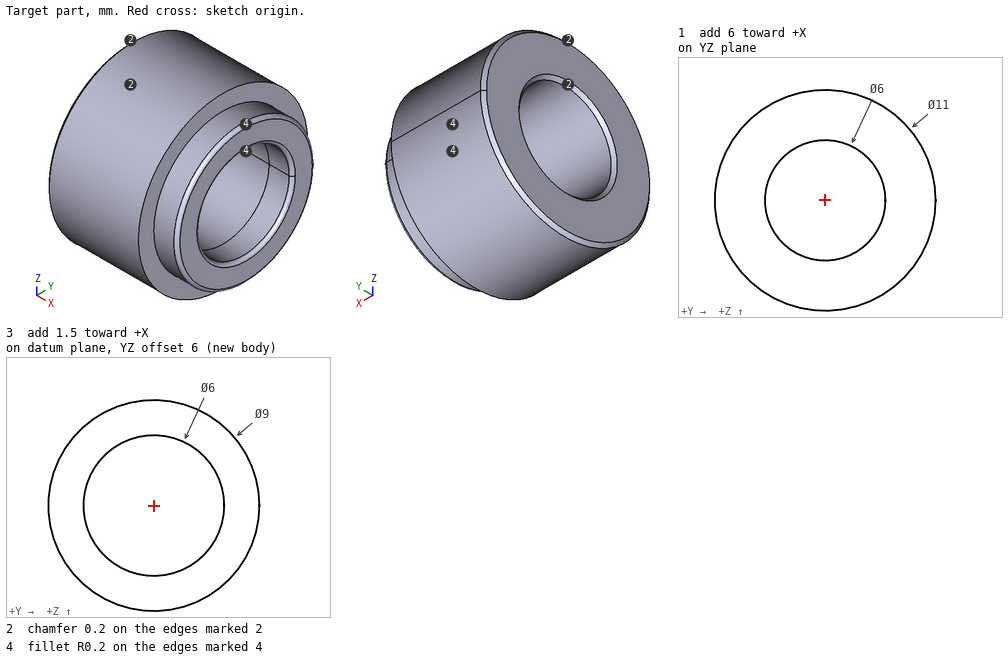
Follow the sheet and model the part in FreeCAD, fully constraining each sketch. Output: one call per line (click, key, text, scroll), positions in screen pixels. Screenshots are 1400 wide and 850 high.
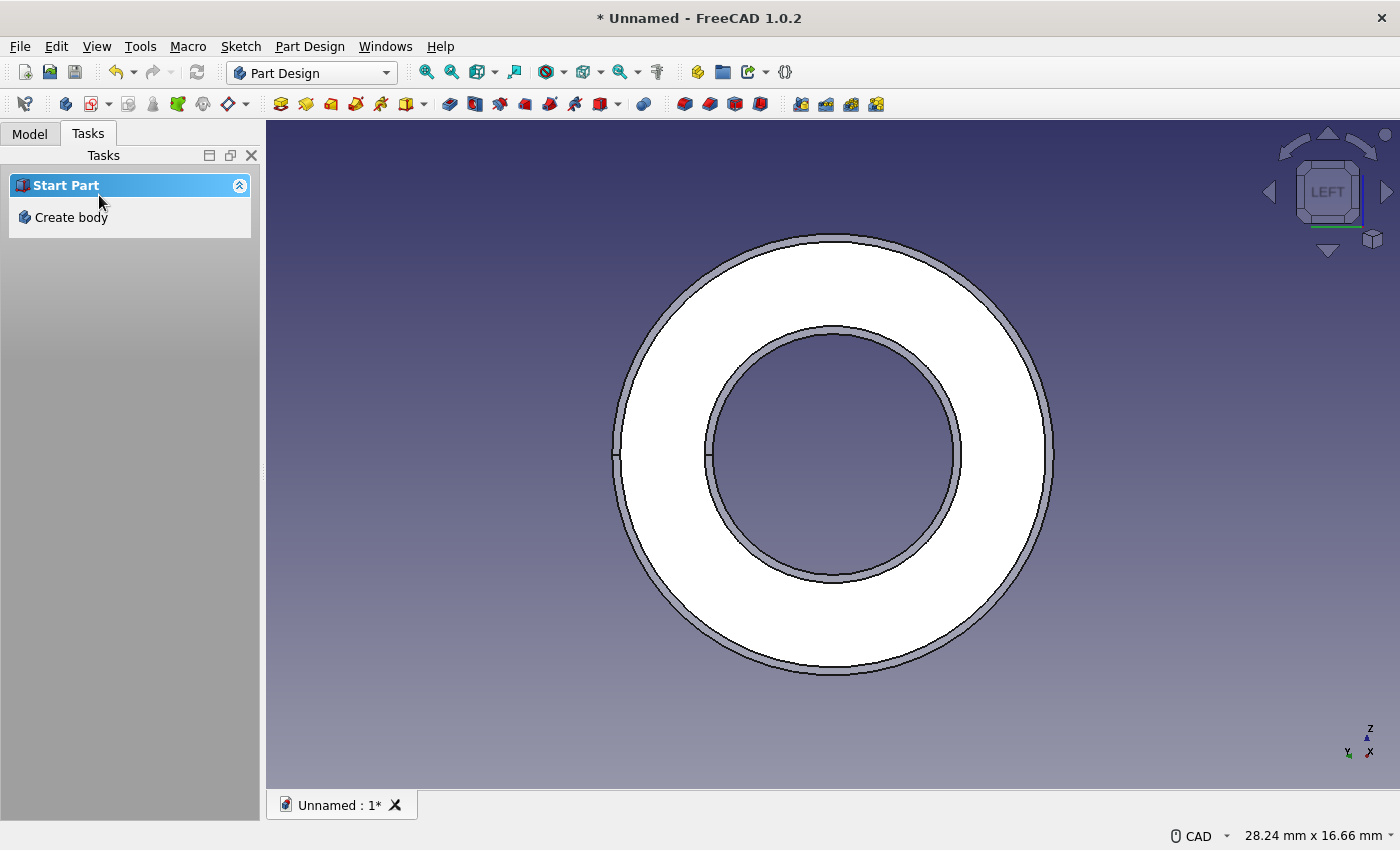
click(66, 104)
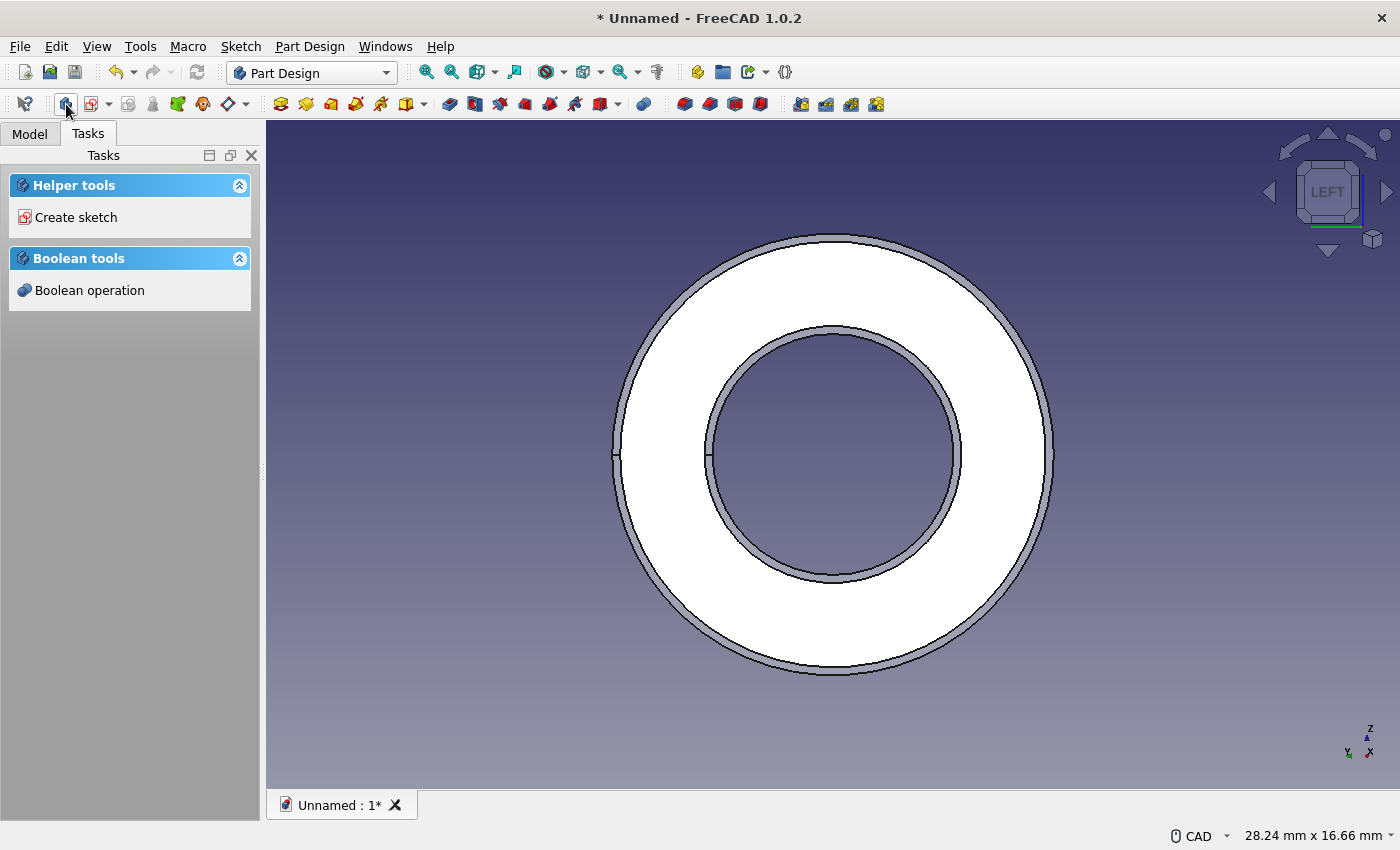
click(30, 134)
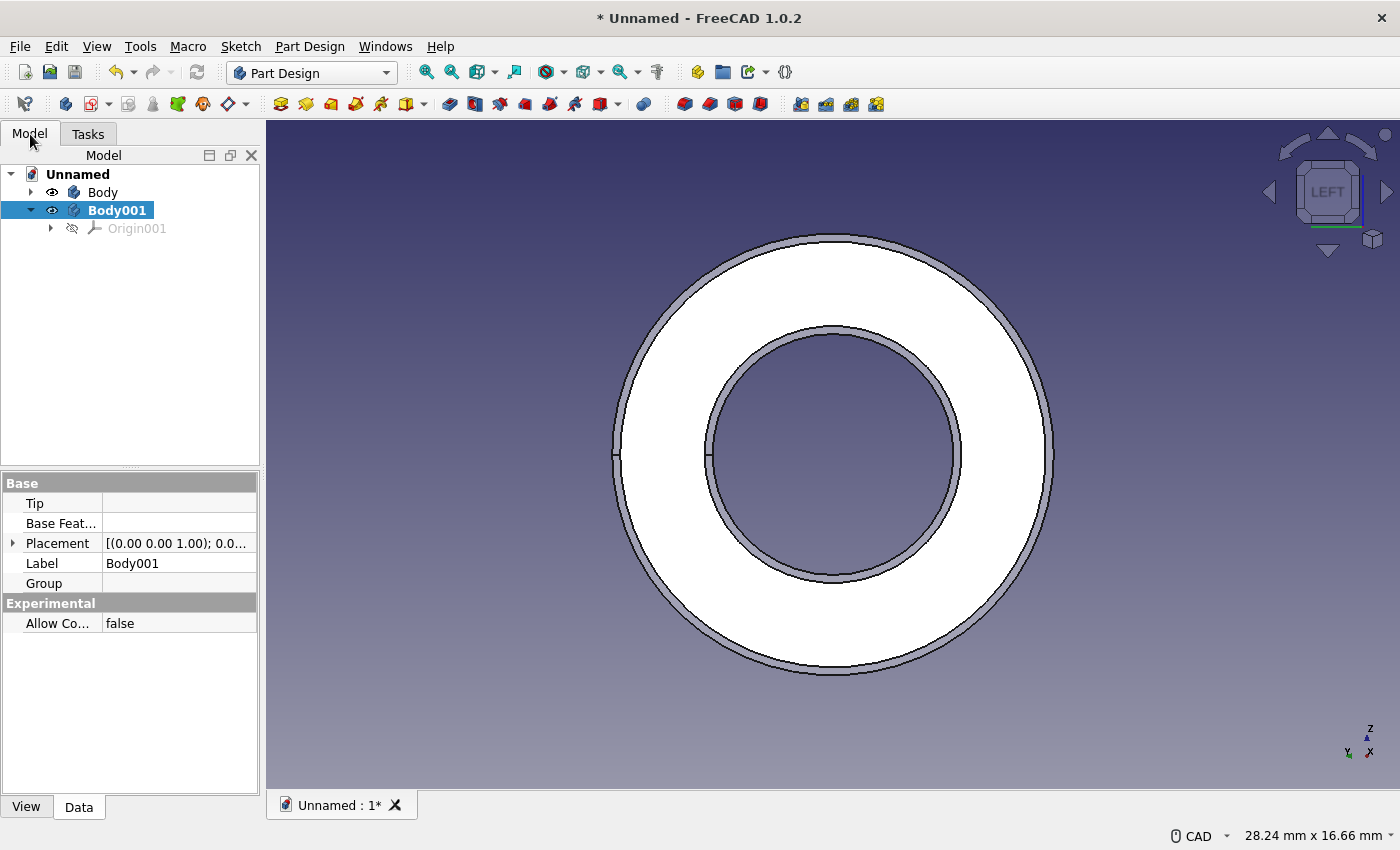
click(51, 228)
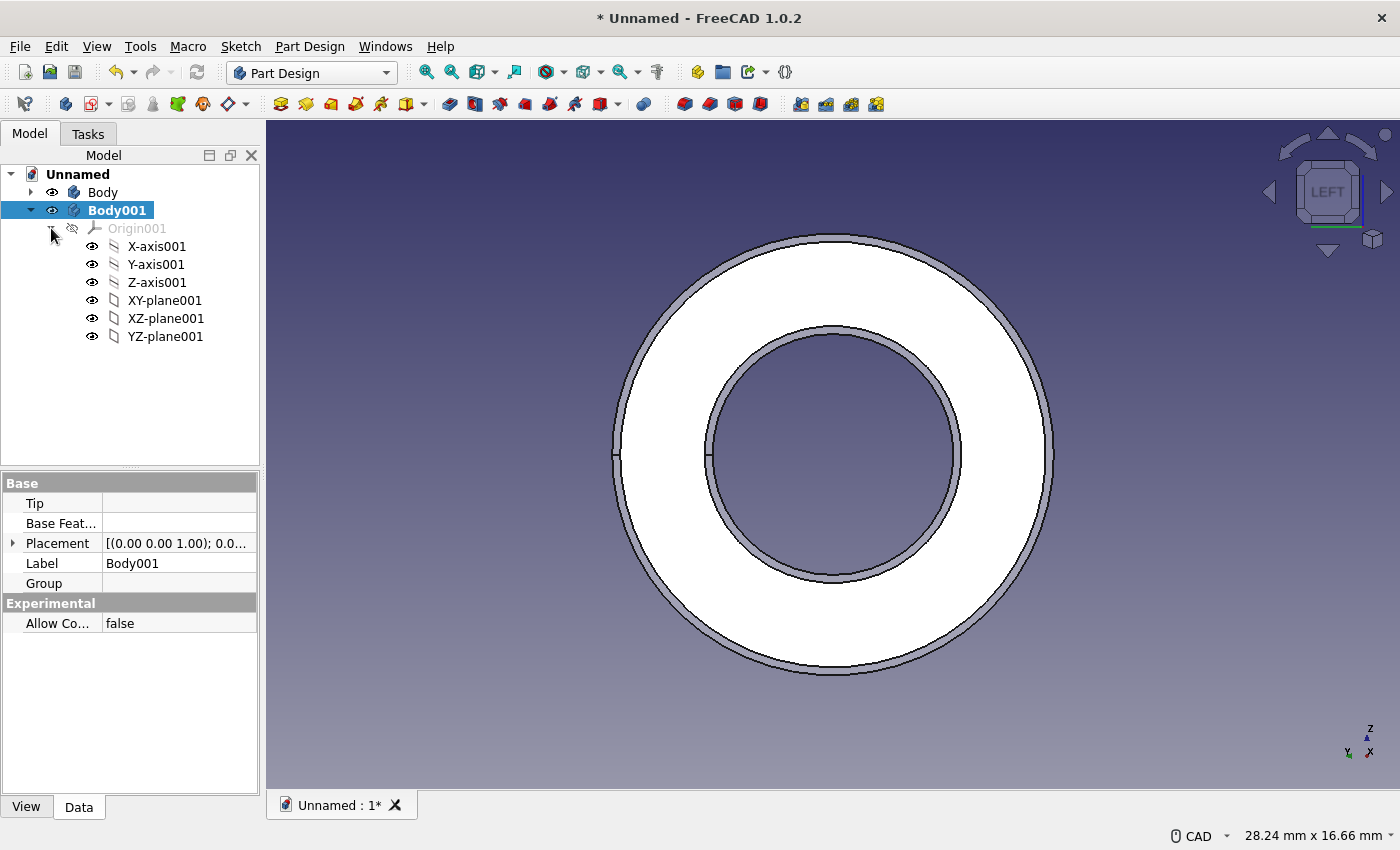
click(137, 336)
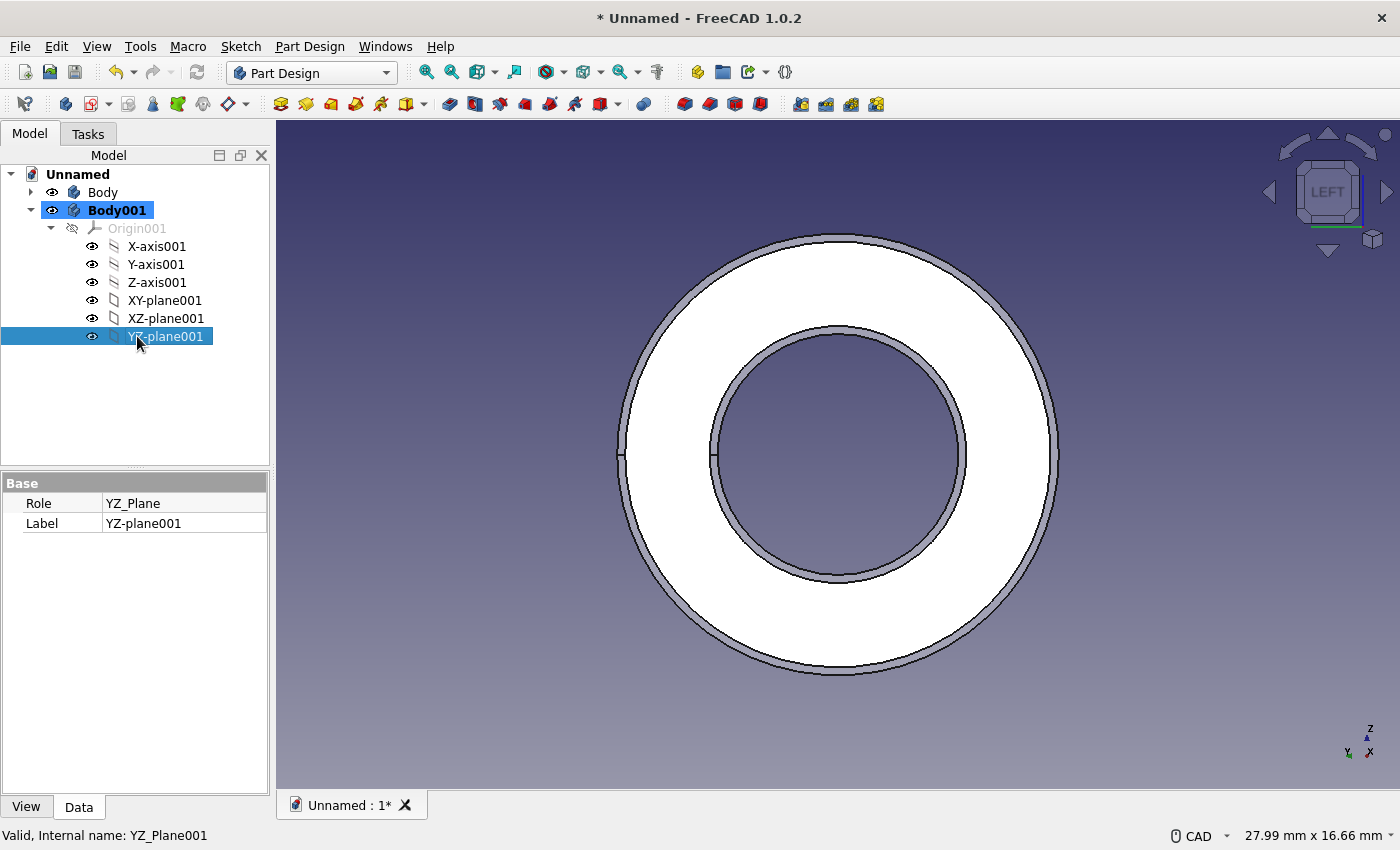
click(228, 104)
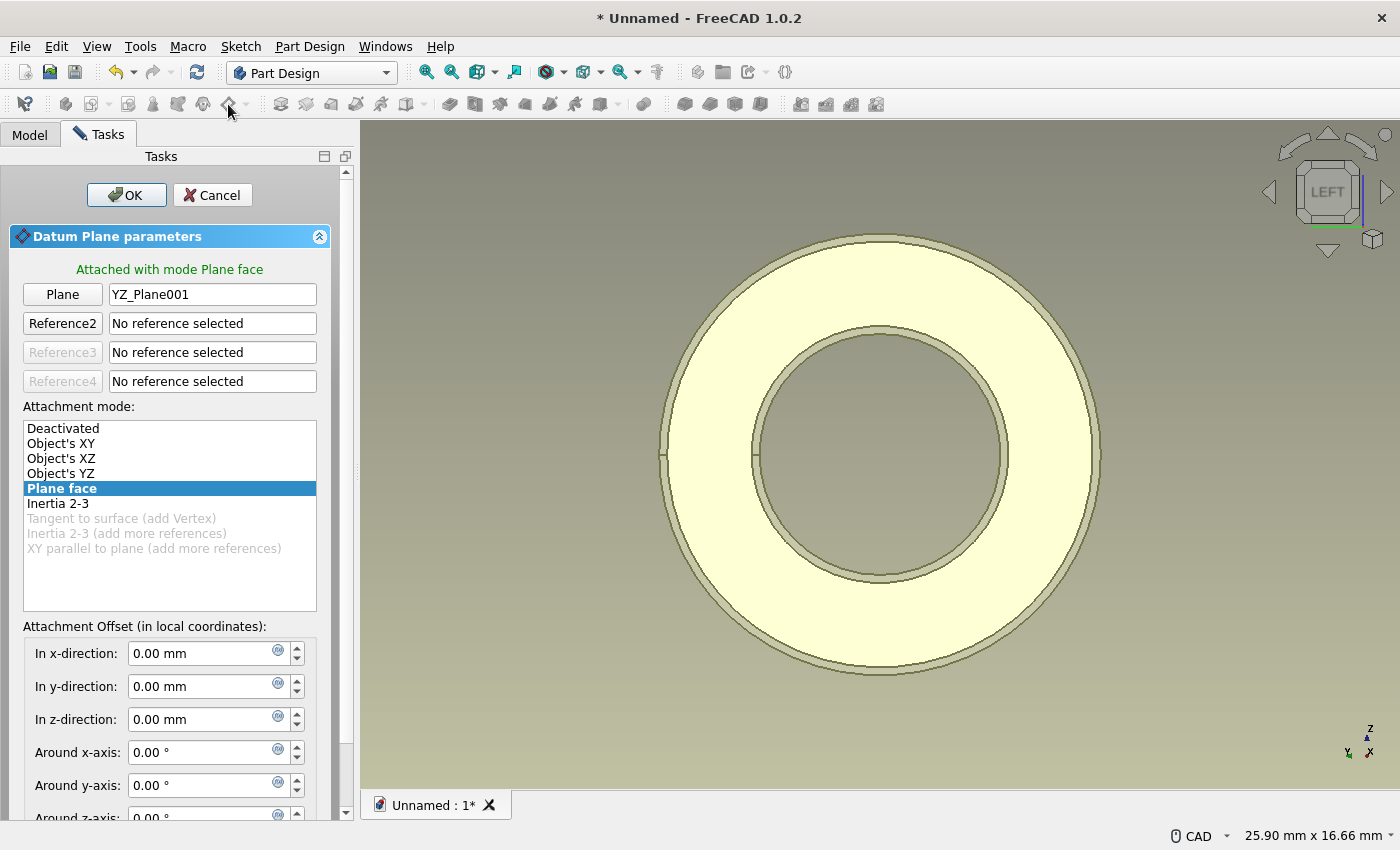
triple_click(210, 720)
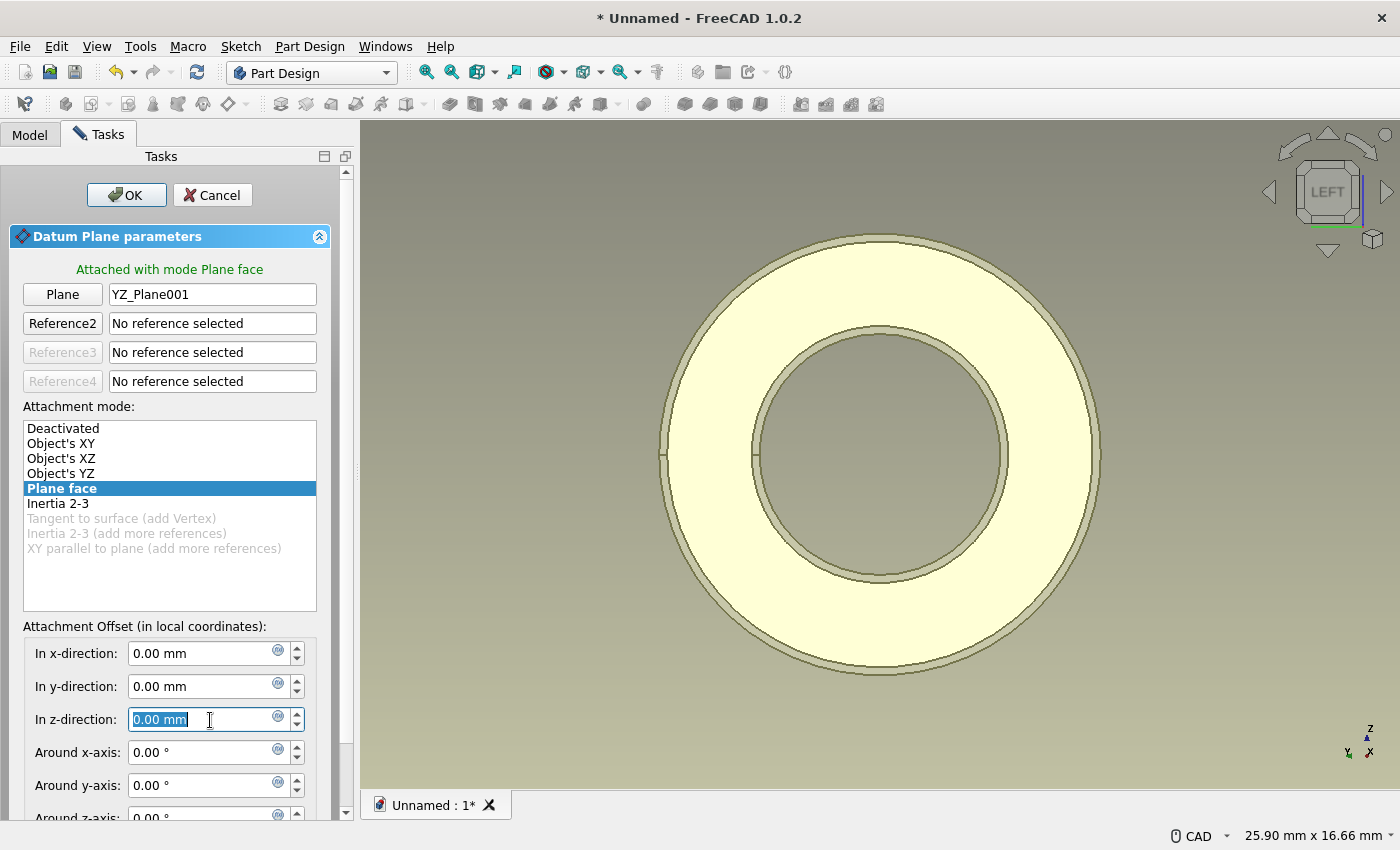
text(6)
key(Tab)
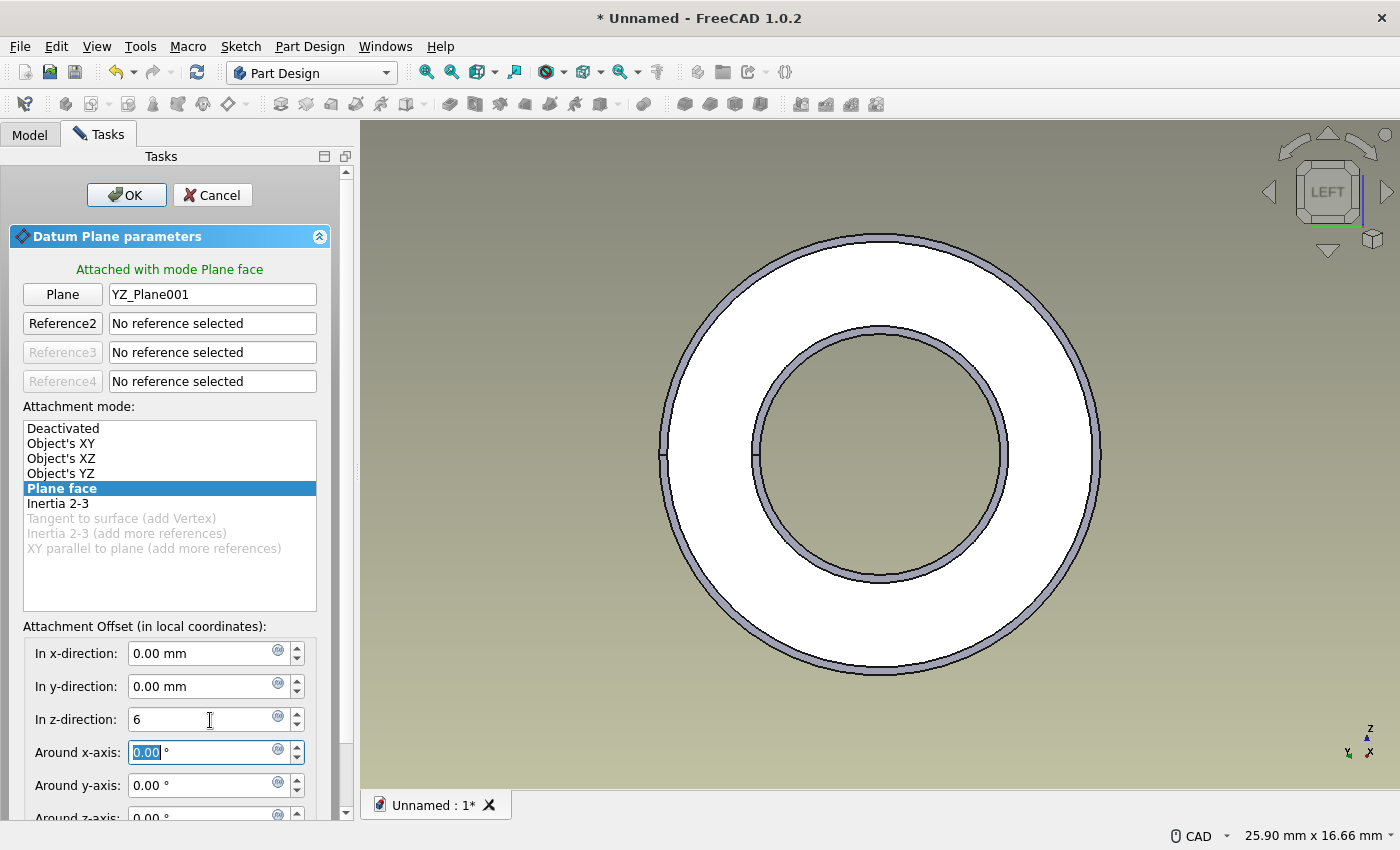
click(127, 195)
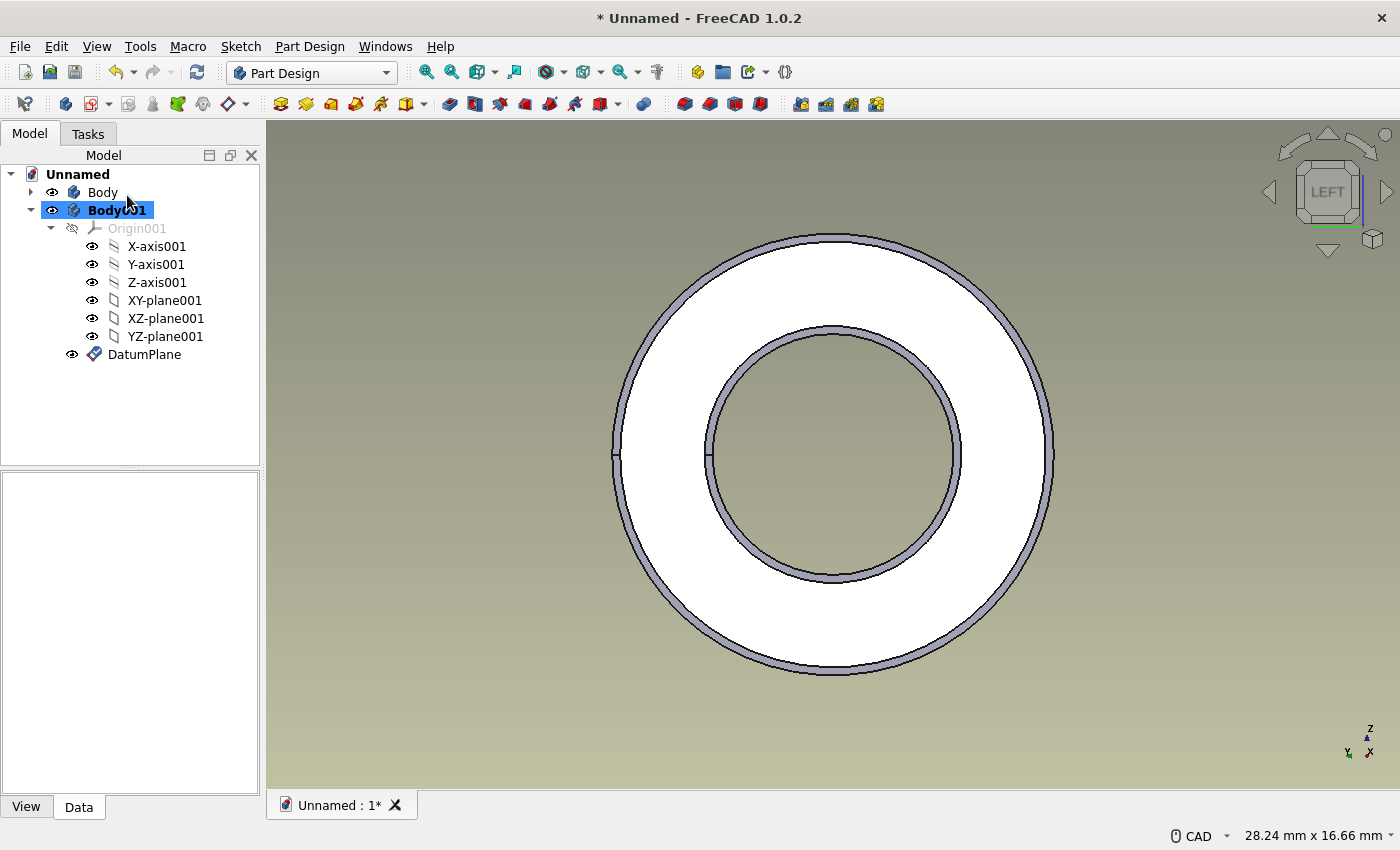
click(117, 354)